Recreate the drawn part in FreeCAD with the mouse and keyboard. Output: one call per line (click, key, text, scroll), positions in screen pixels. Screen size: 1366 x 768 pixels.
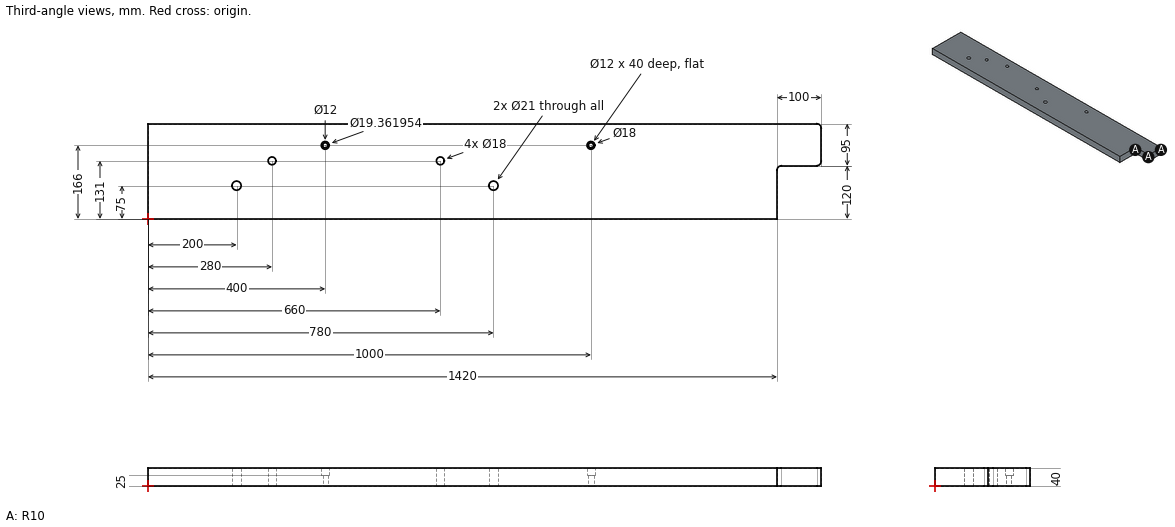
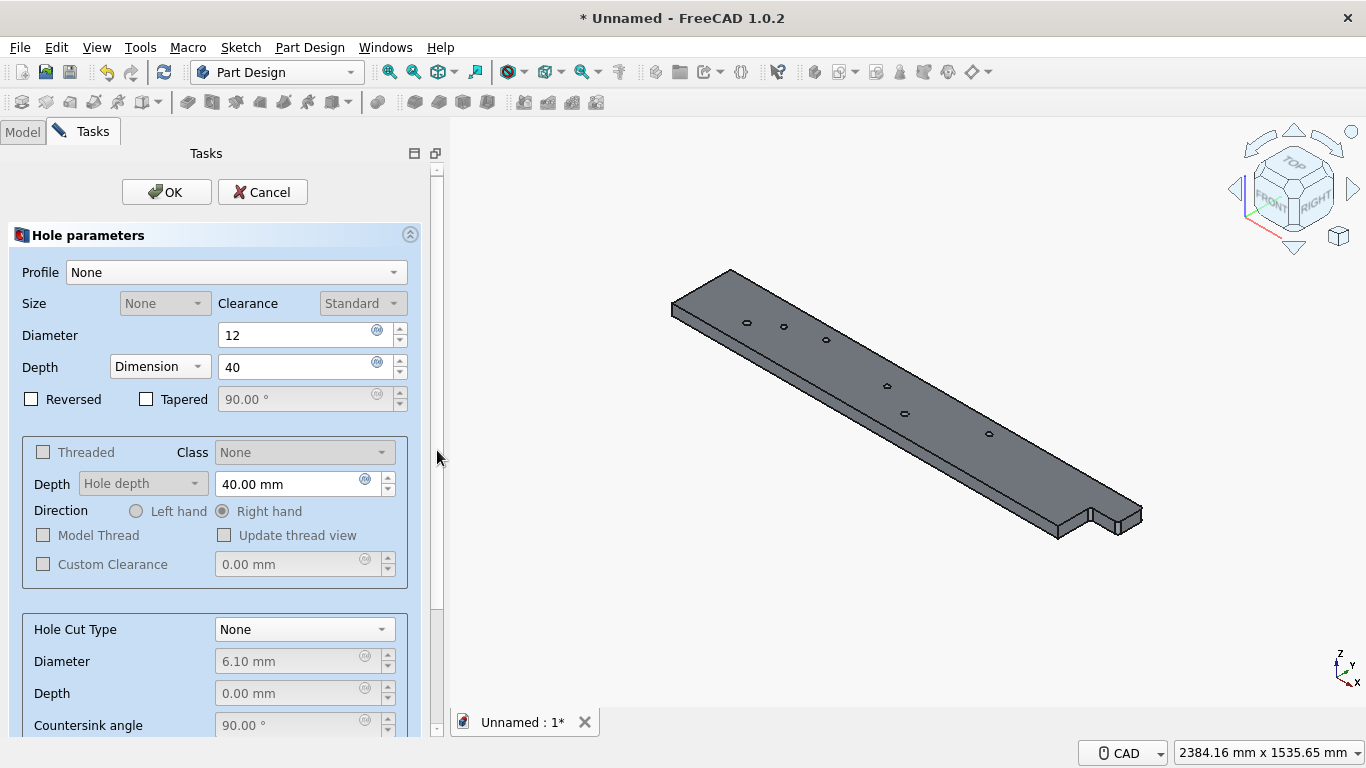
click(167, 192)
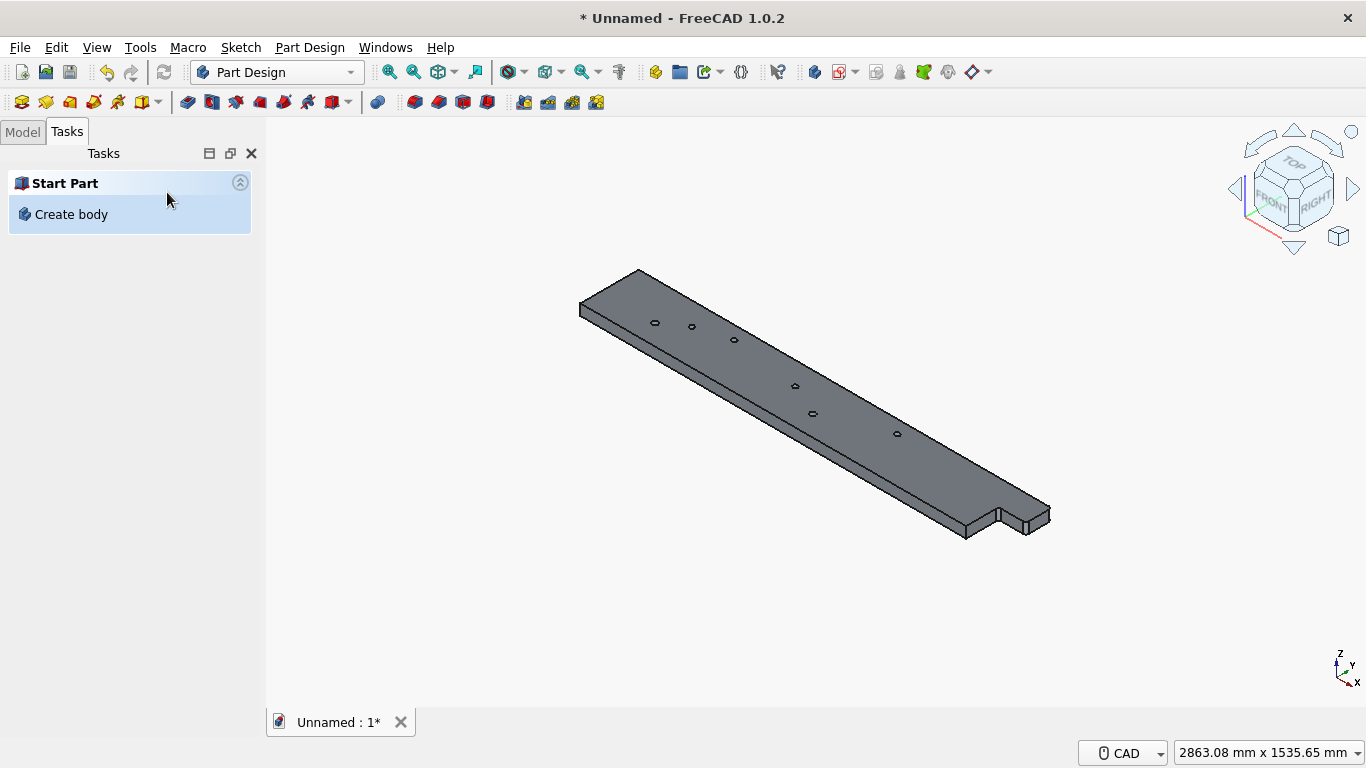
scroll(734, 344, up, 7)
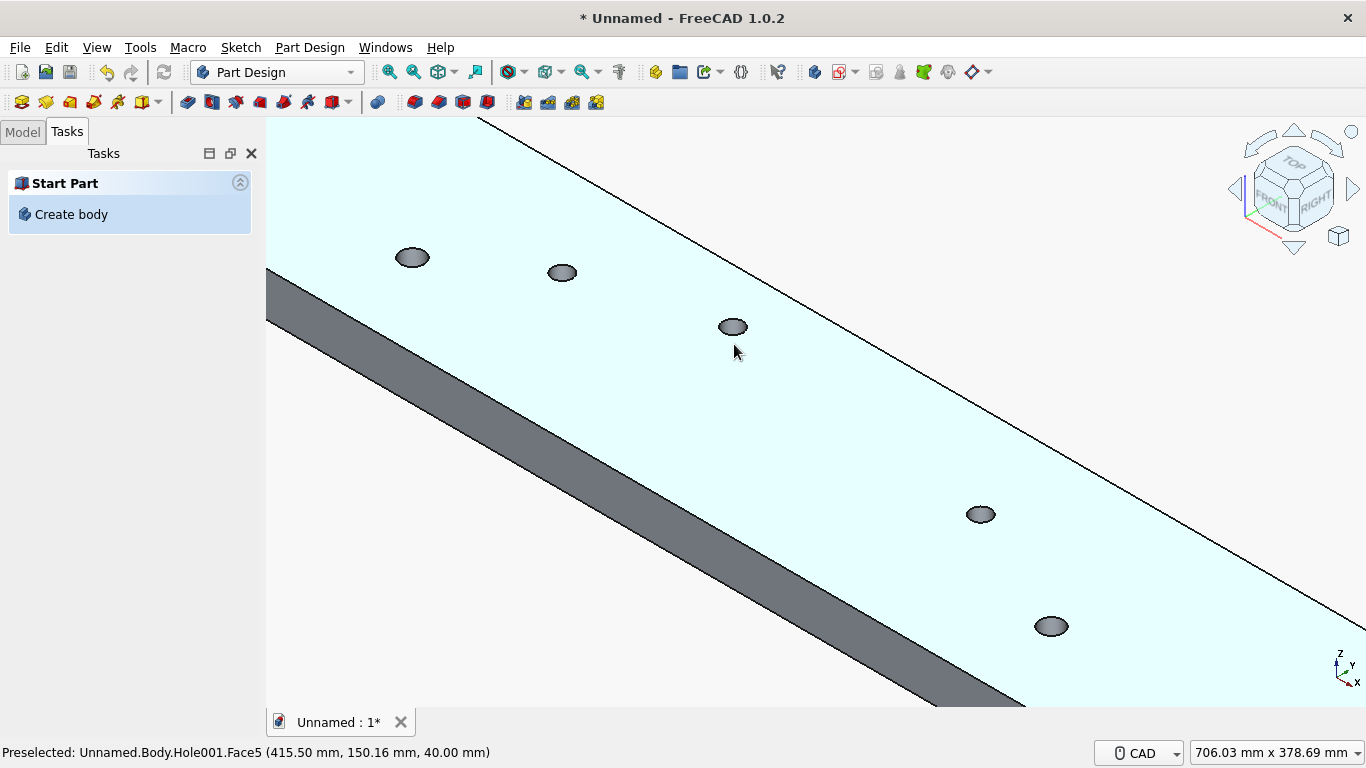
key(v)
key(f)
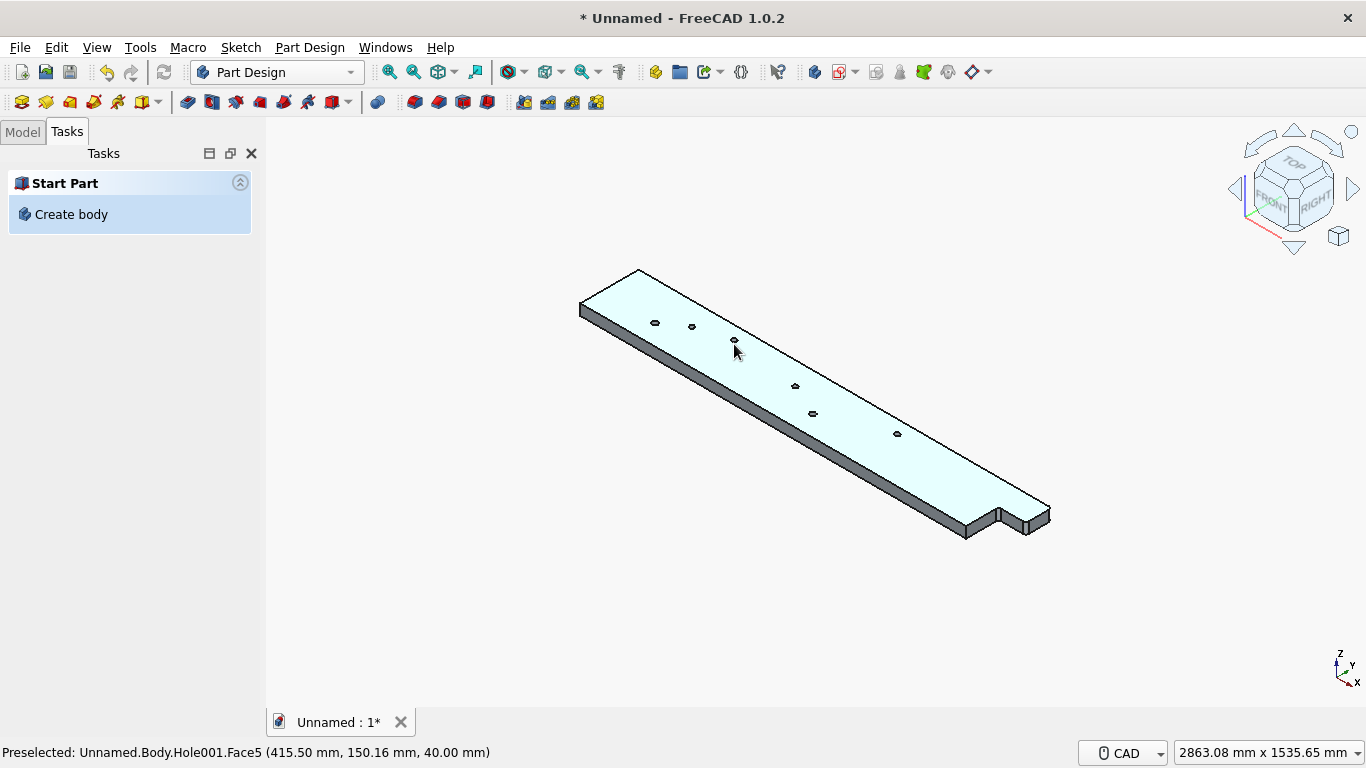
key(2)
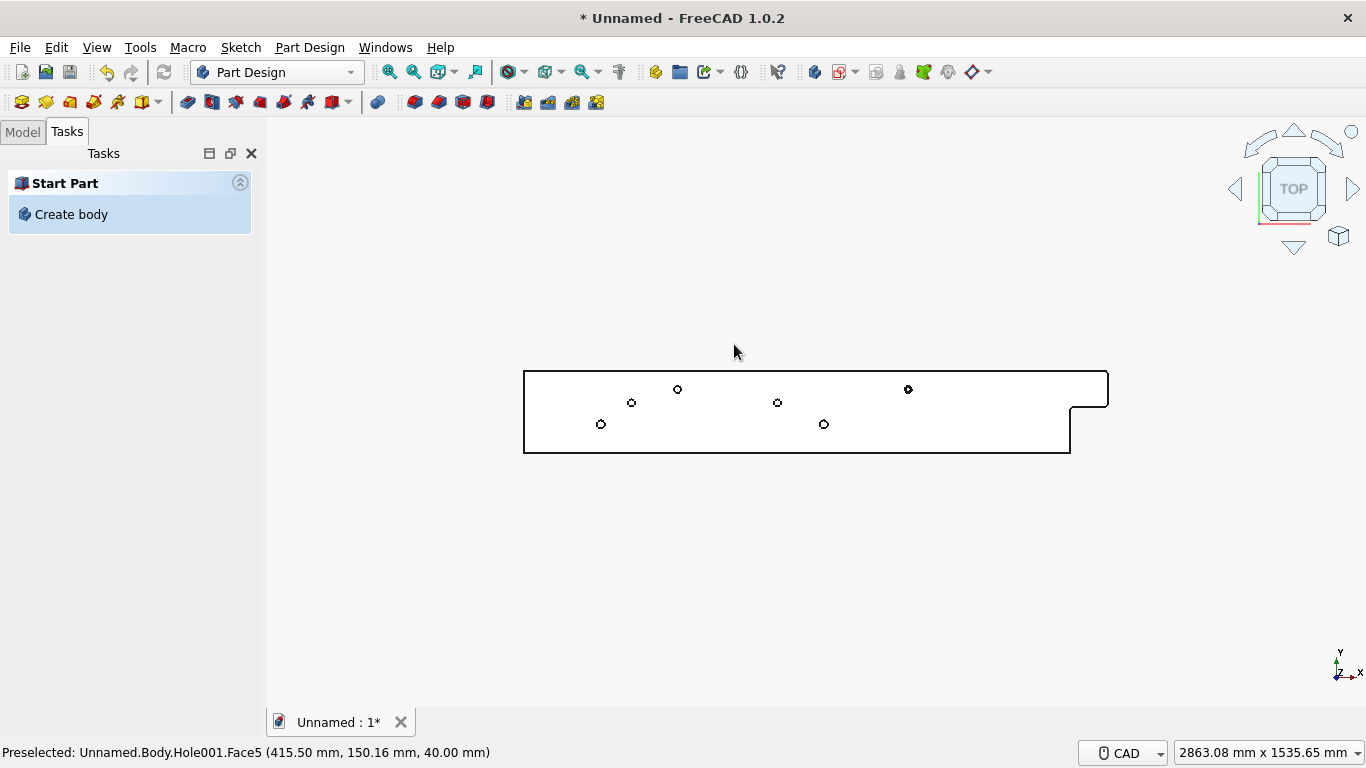
scroll(678, 389, up, 7)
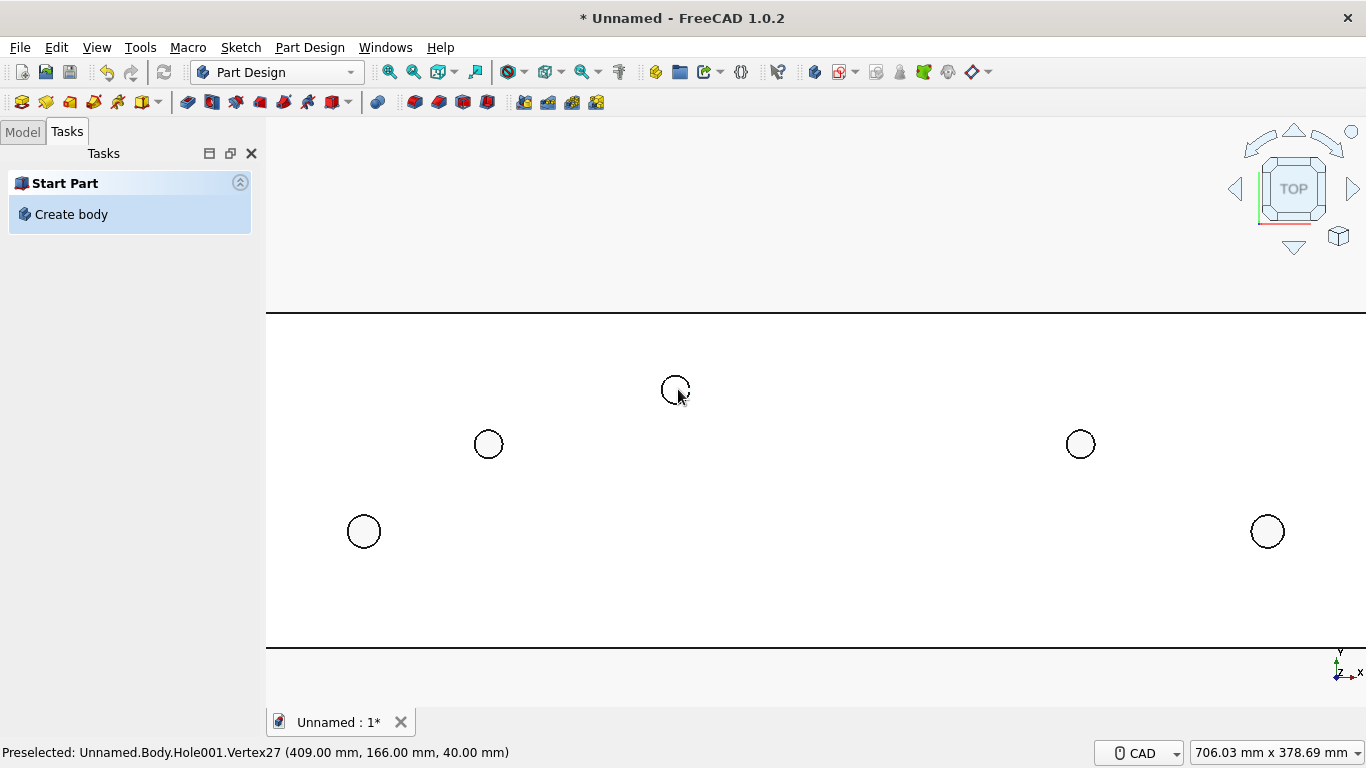
click(676, 389)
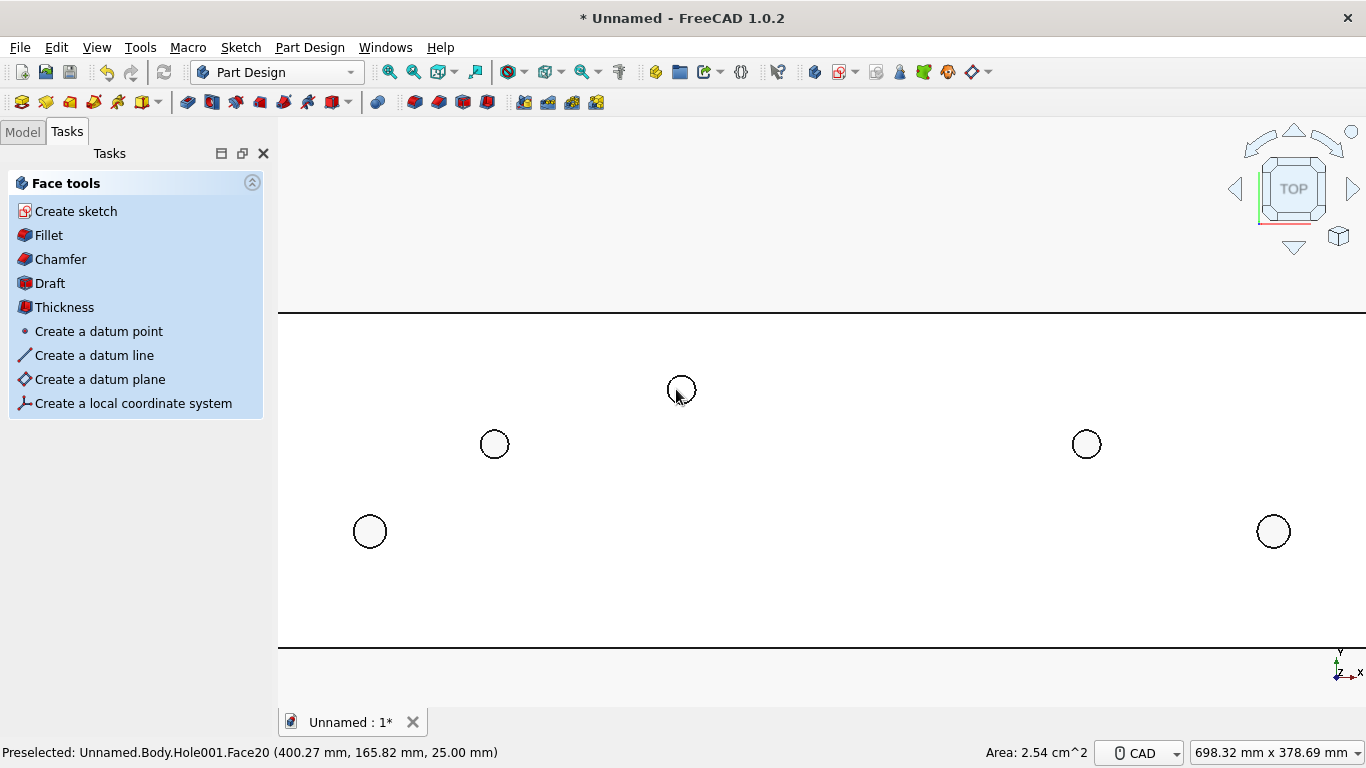
click(840, 72)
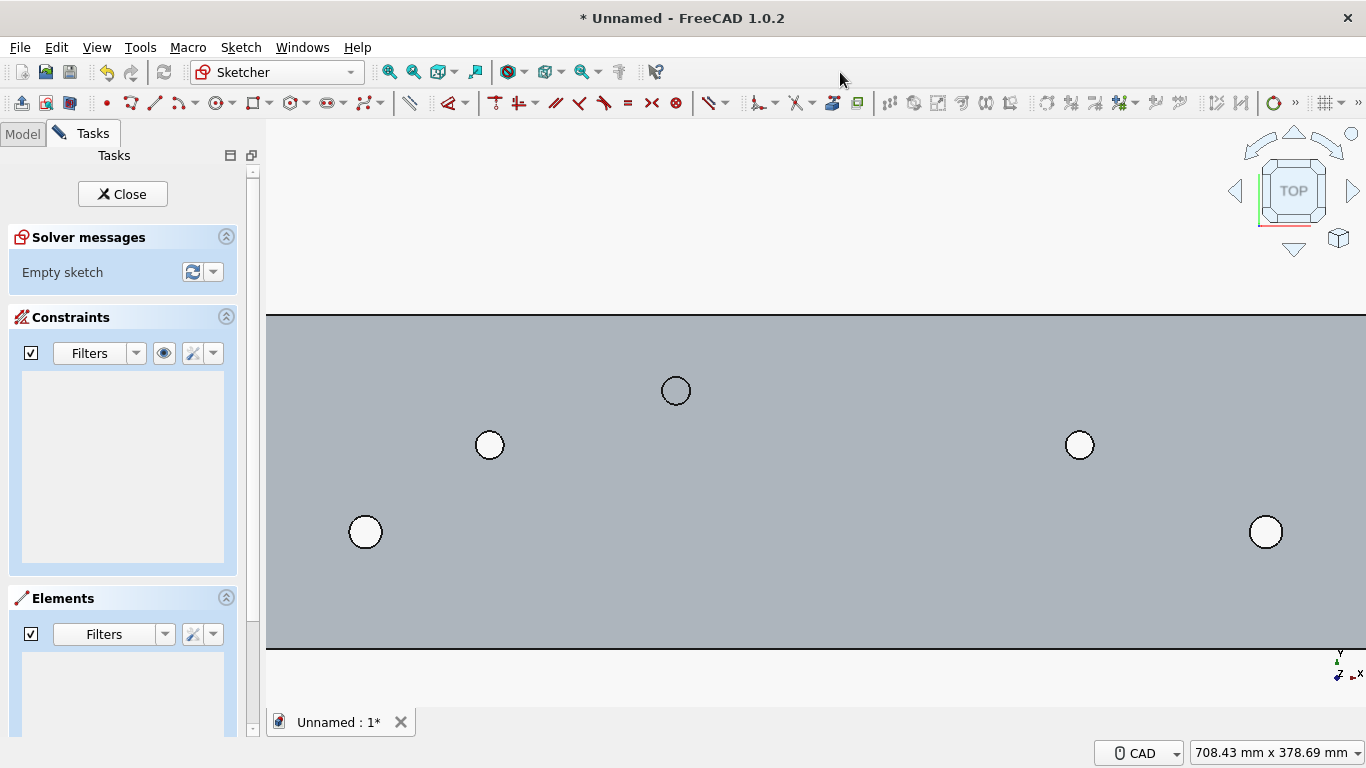
click(70, 104)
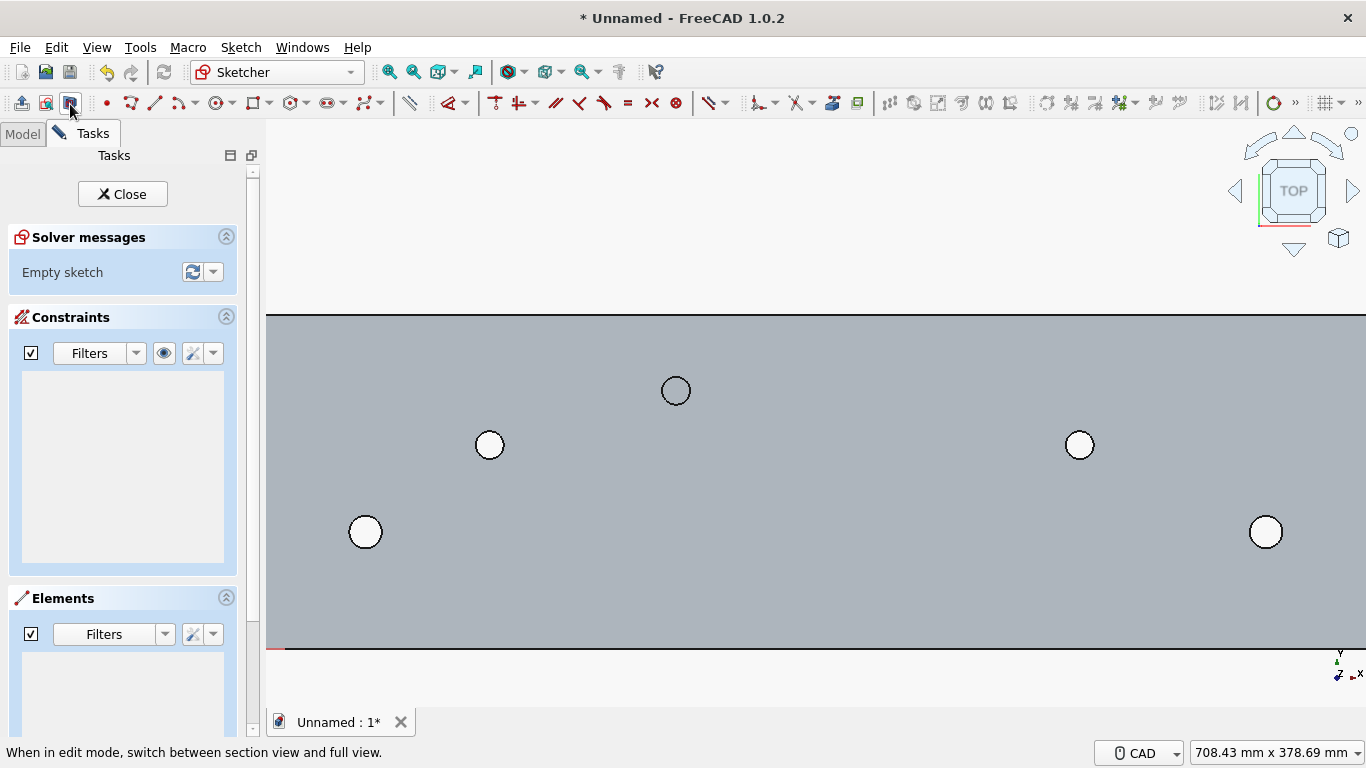
scroll(672, 390, up, 15)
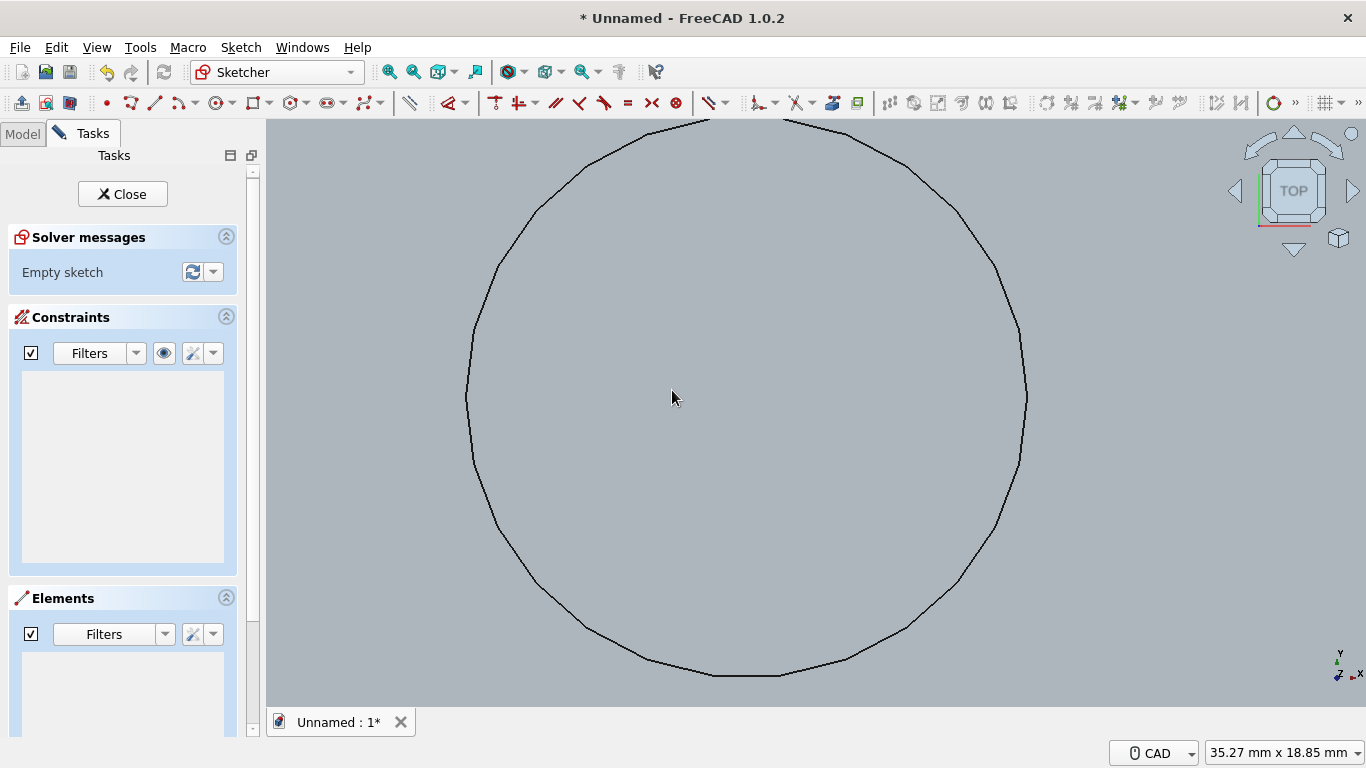
key(g)
key(c)